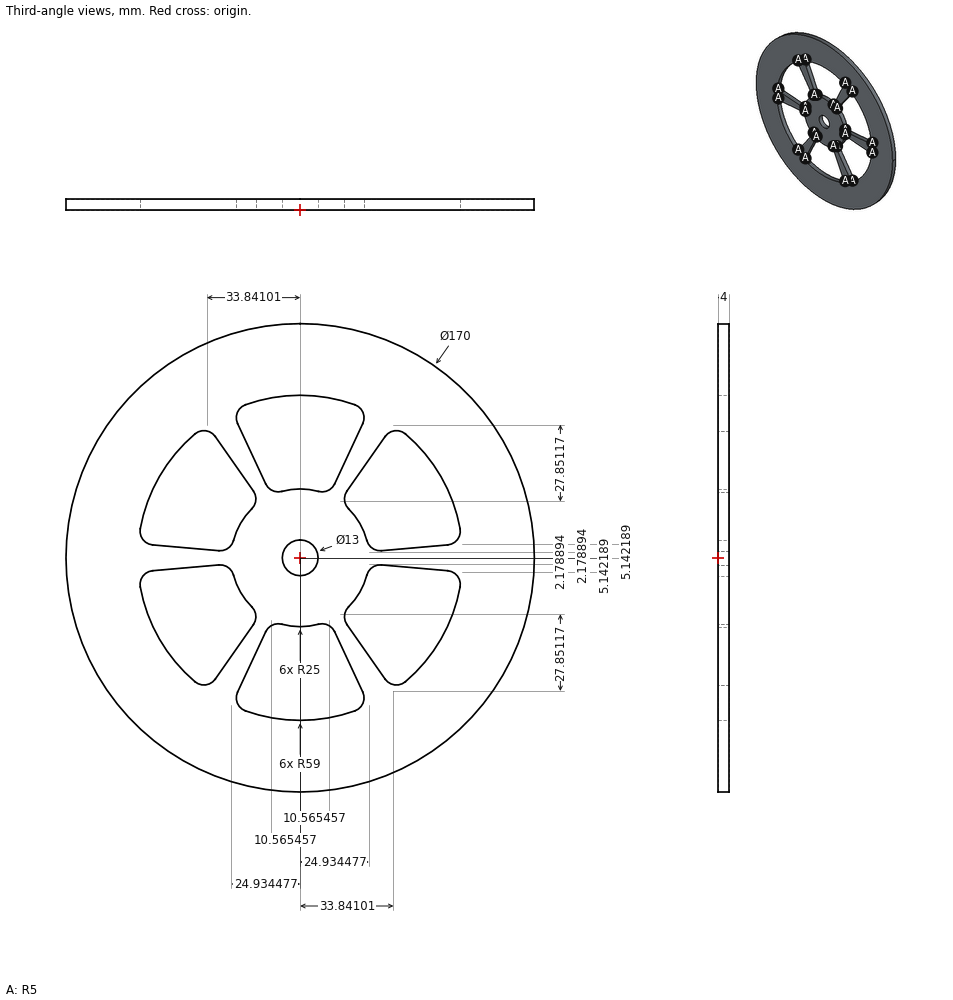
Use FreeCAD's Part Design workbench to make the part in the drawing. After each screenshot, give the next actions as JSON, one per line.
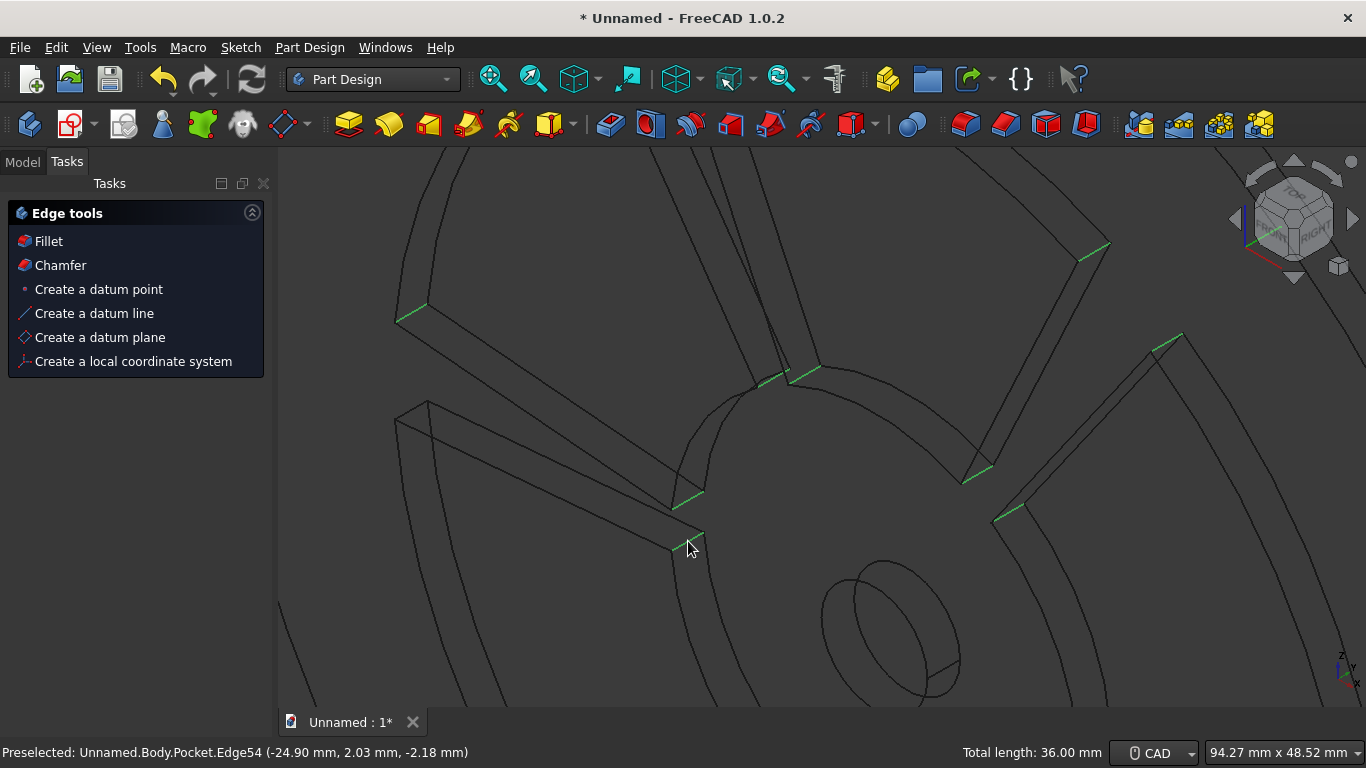
{"action": "left_click", "coordinate": [411, 409], "text": "ctrl"}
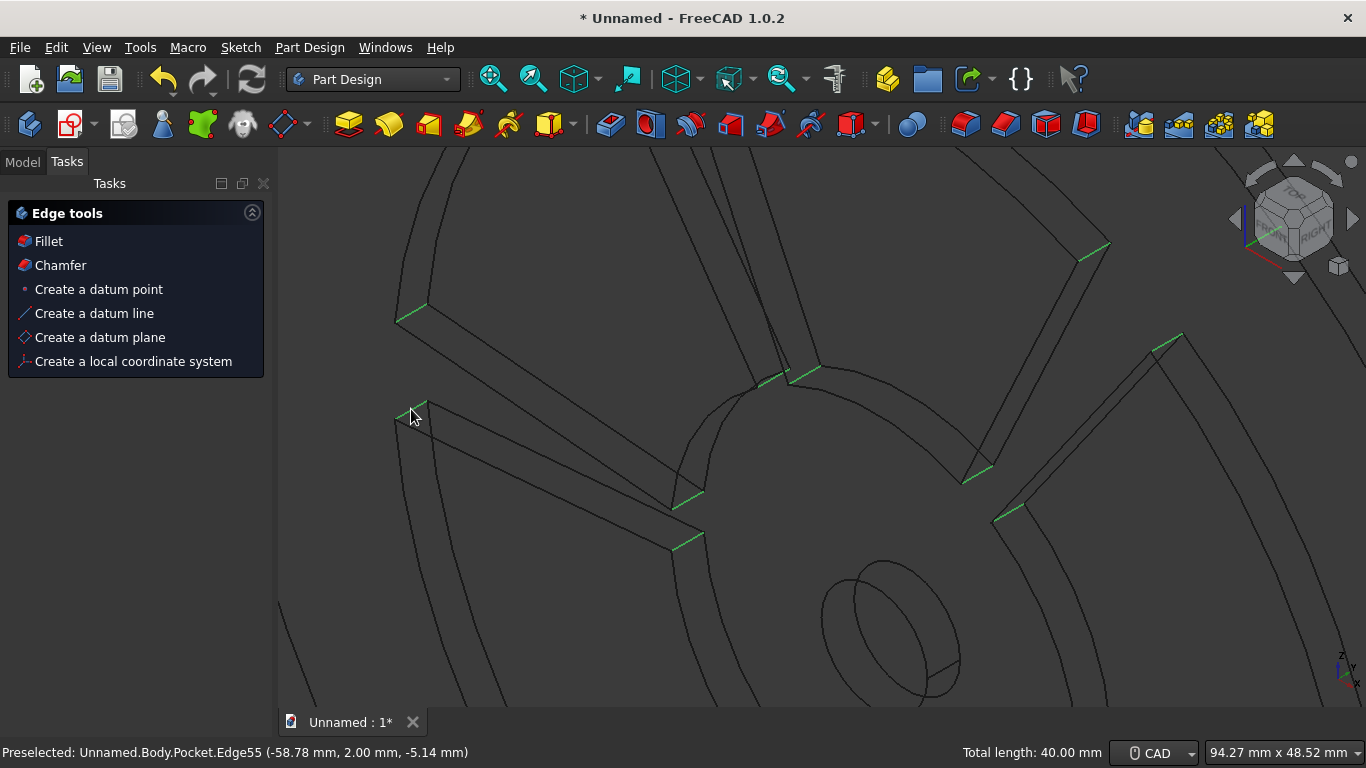
{"action": "left_click", "coordinate": [494, 80]}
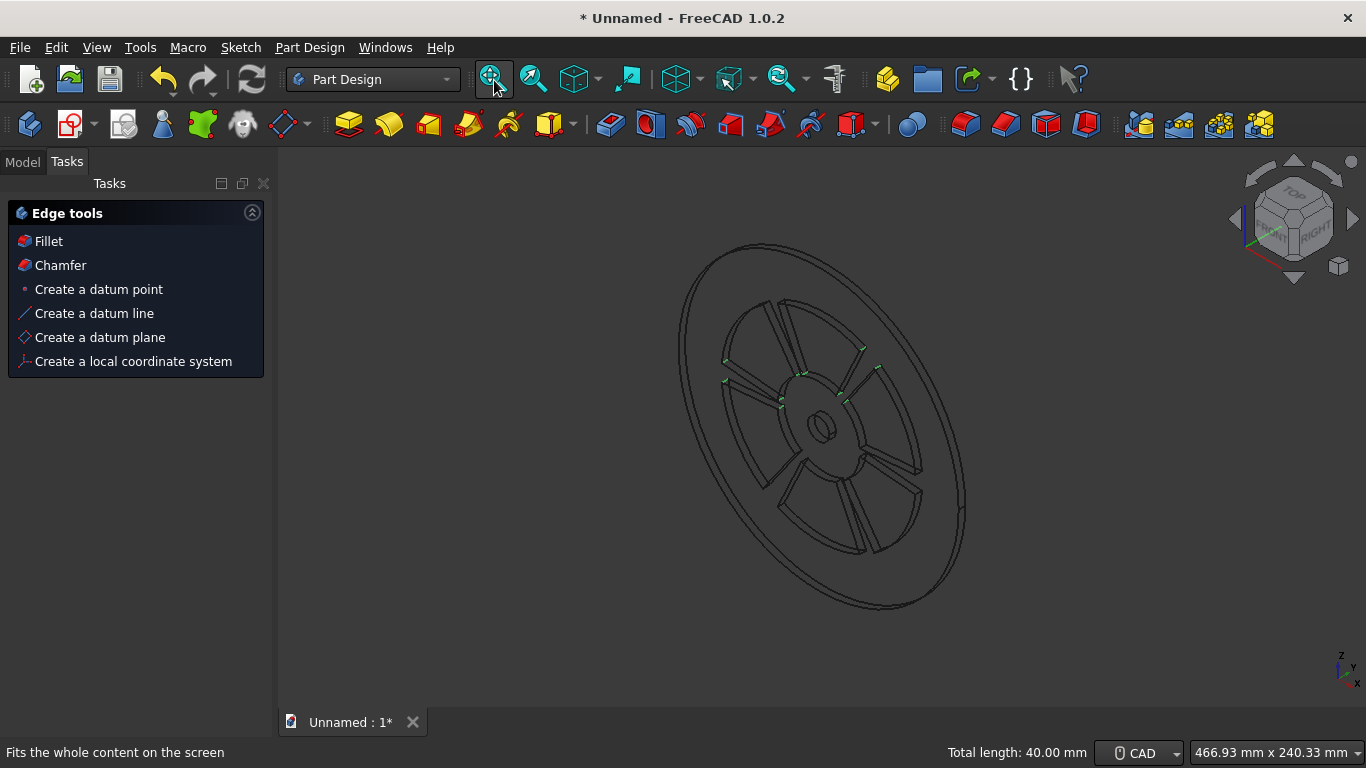
{"action": "key", "text": "2"}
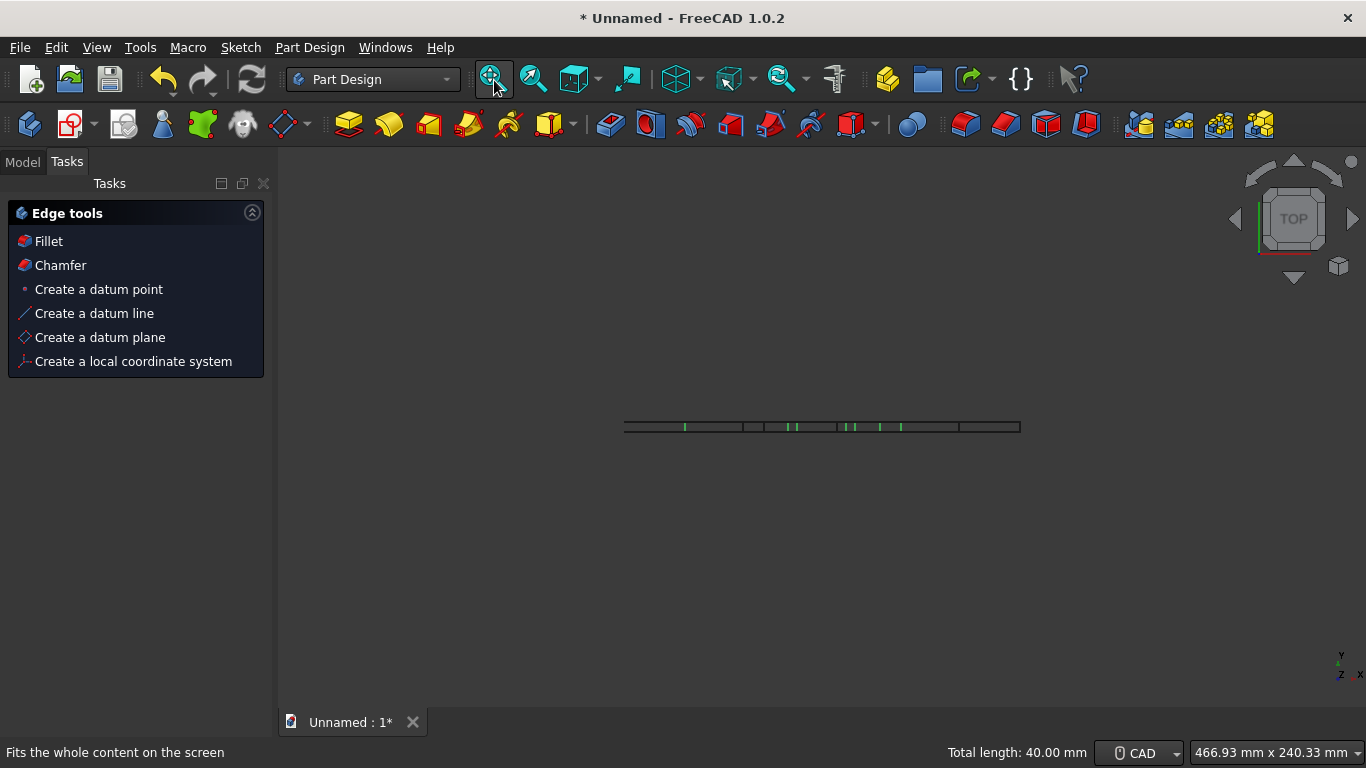
{"action": "left_click", "coordinate": [494, 80]}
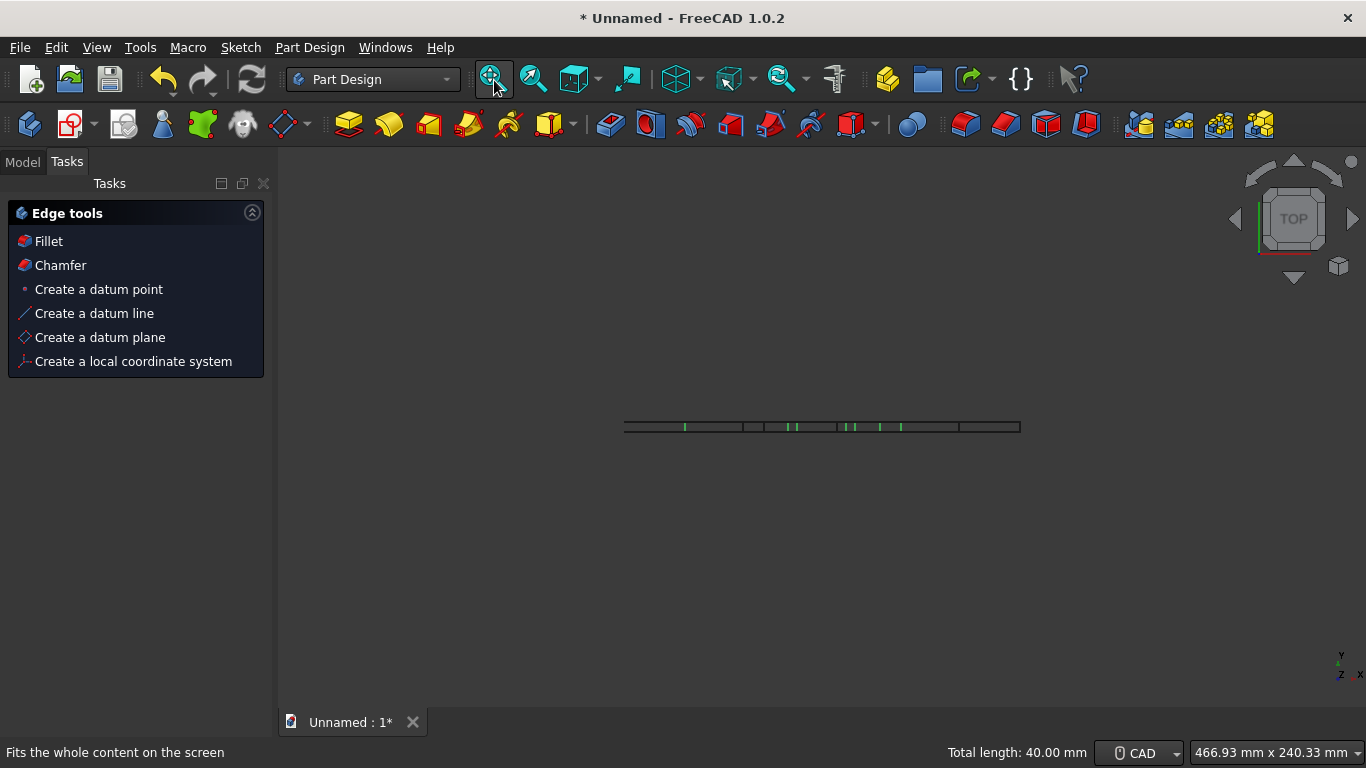
{"action": "scroll", "coordinate": [764, 426], "scroll_direction": "up", "scroll_amount": 8}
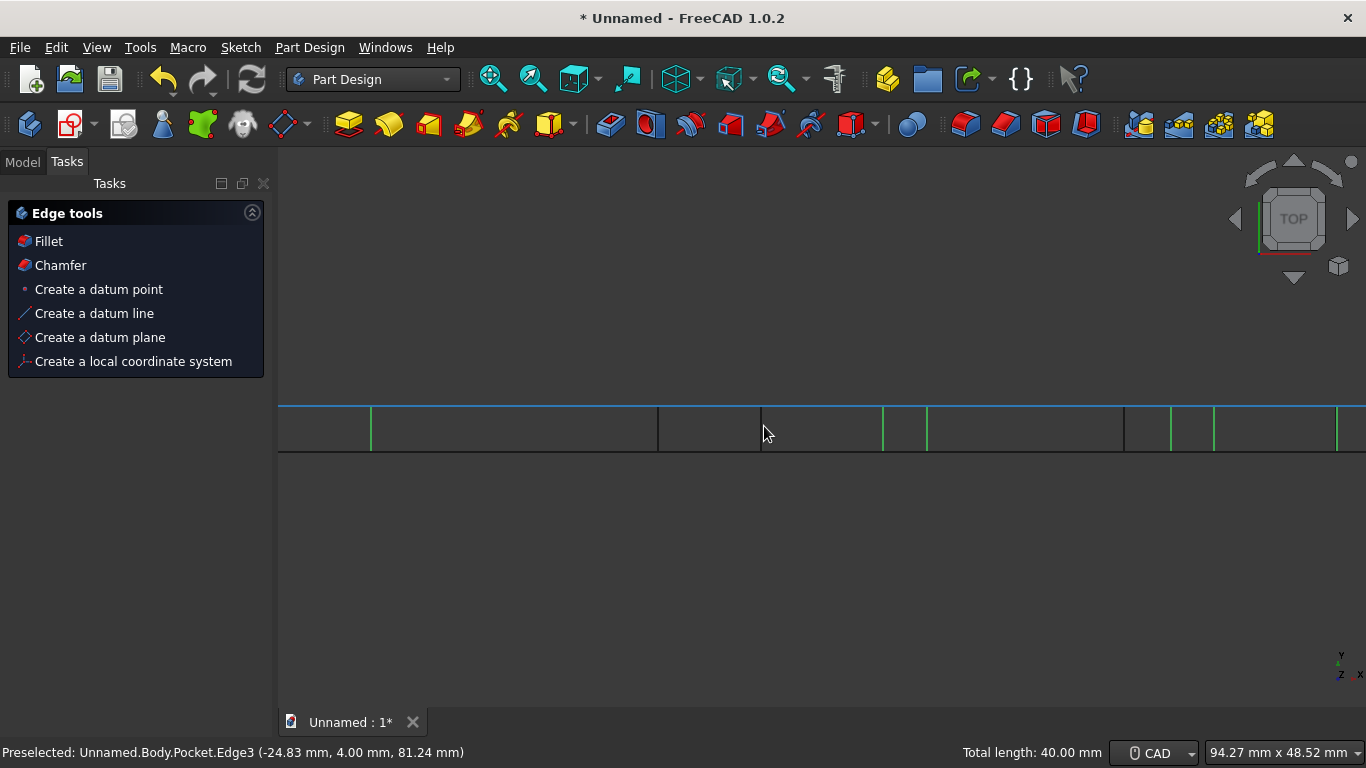
{"action": "left_click", "coordinate": [761, 428], "text": "ctrl"}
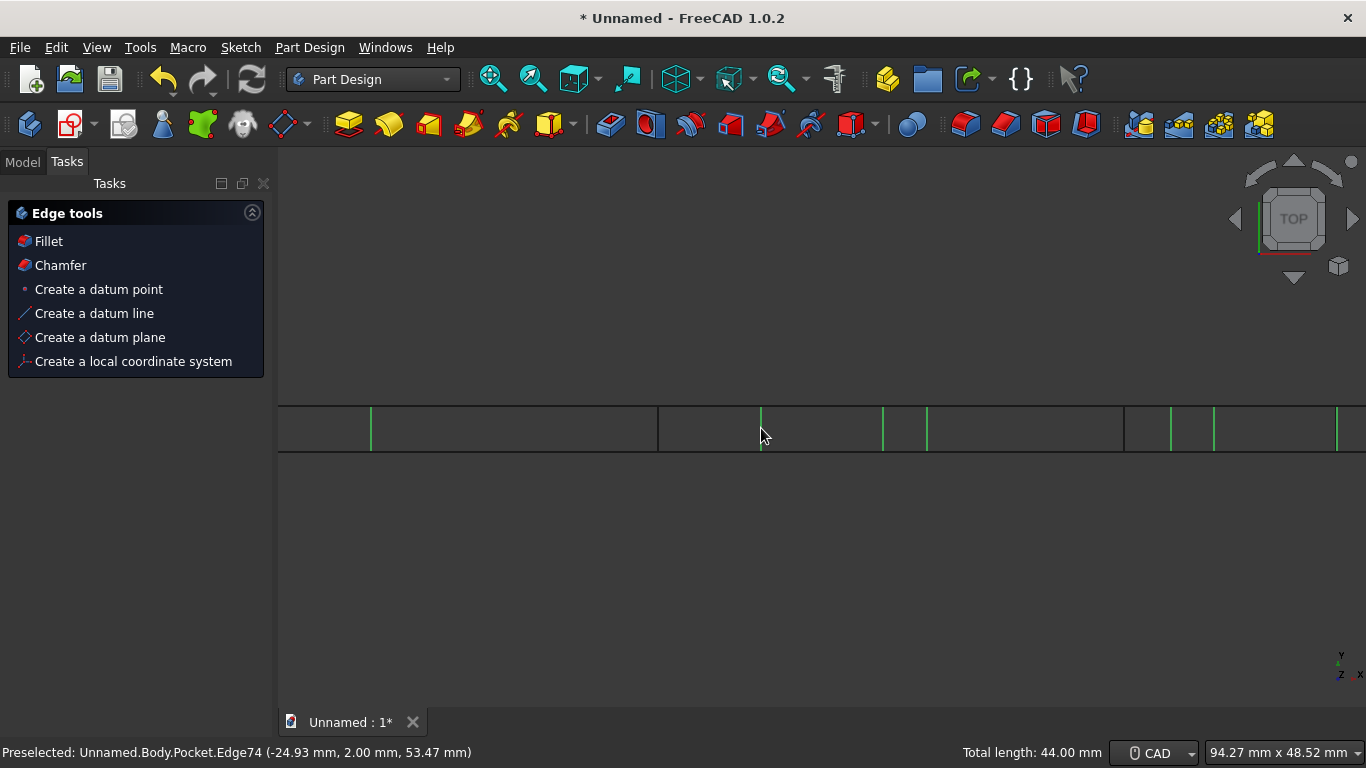
{"action": "left_click", "coordinate": [658, 428], "text": "ctrl"}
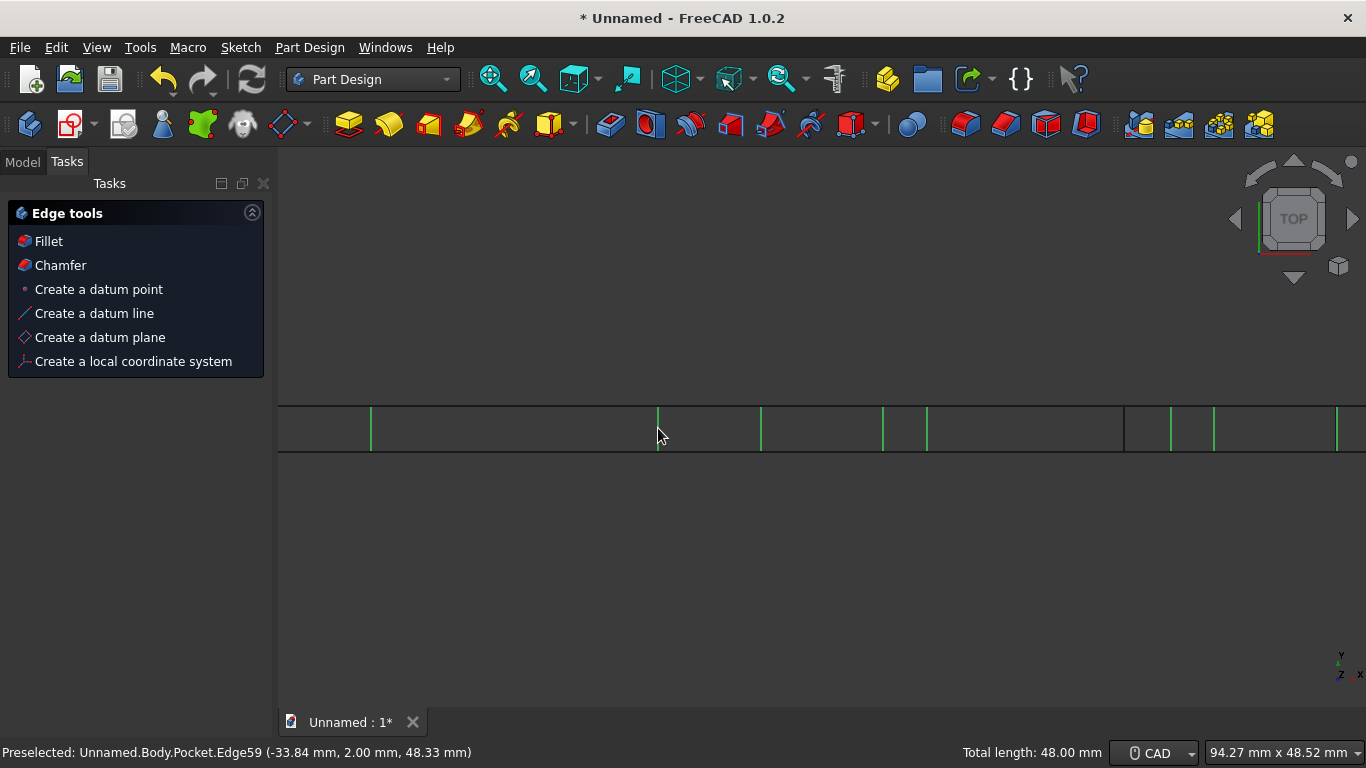
{"action": "left_click", "coordinate": [494, 80]}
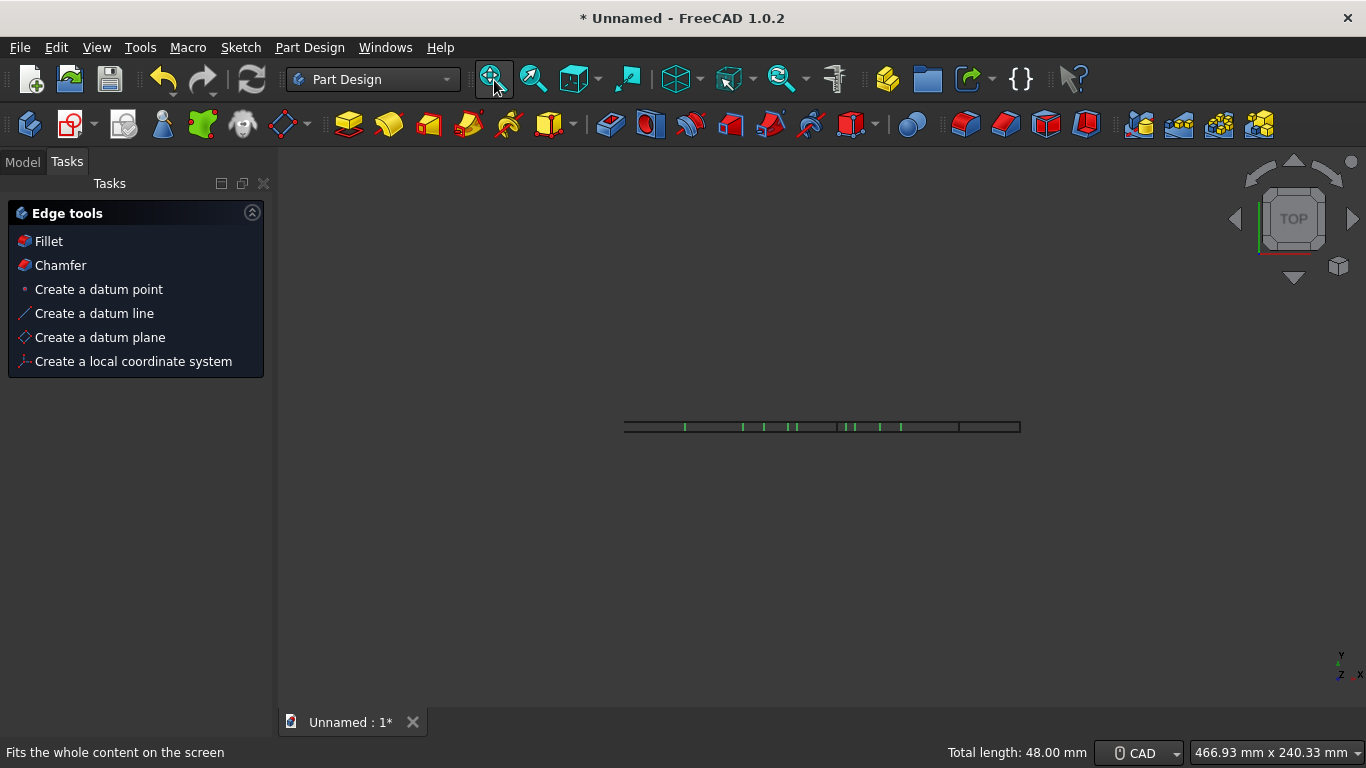
{"action": "key", "text": "1"}